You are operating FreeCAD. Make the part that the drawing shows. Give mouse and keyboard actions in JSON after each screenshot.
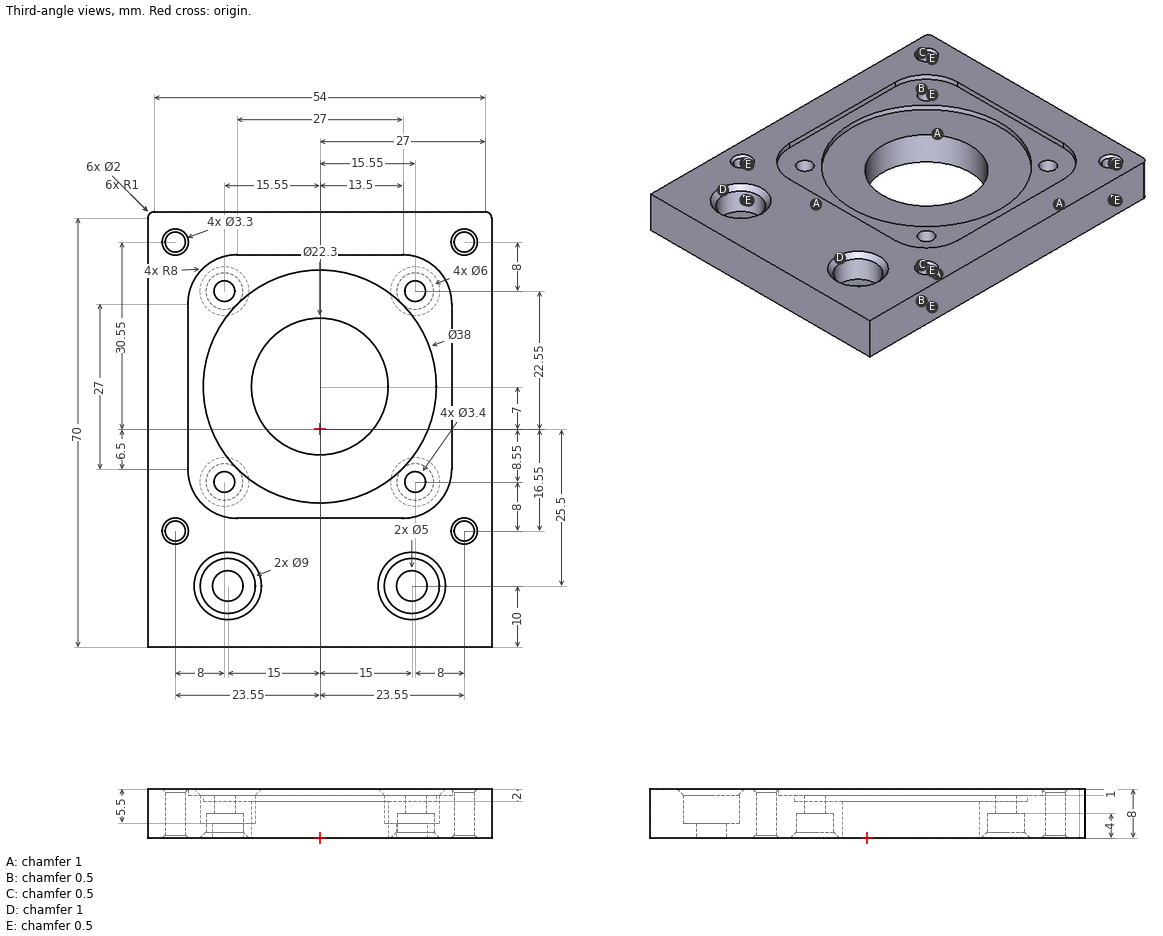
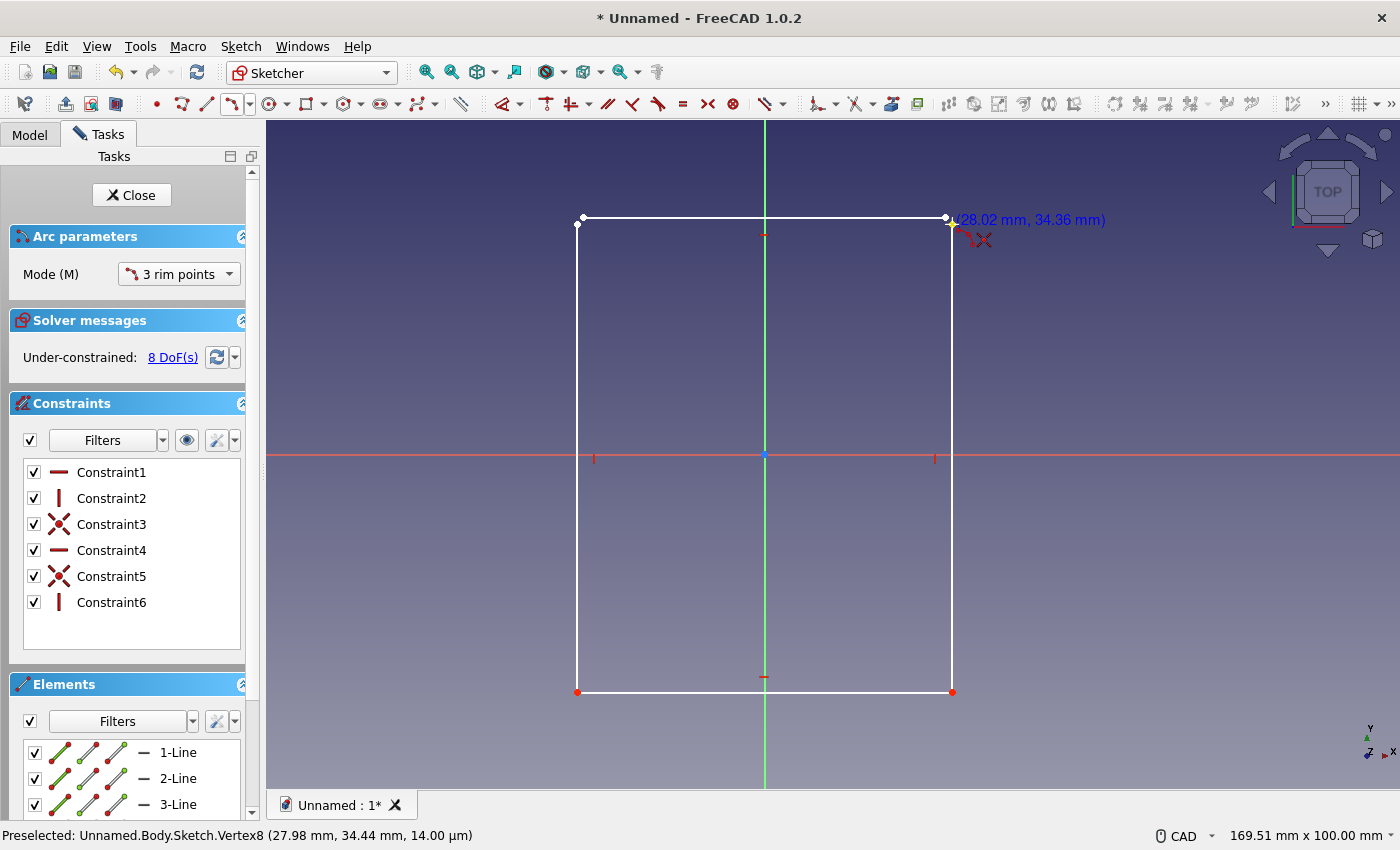
{"action": "scroll", "coordinate": [584, 217], "scroll_direction": "up", "scroll_amount": 3}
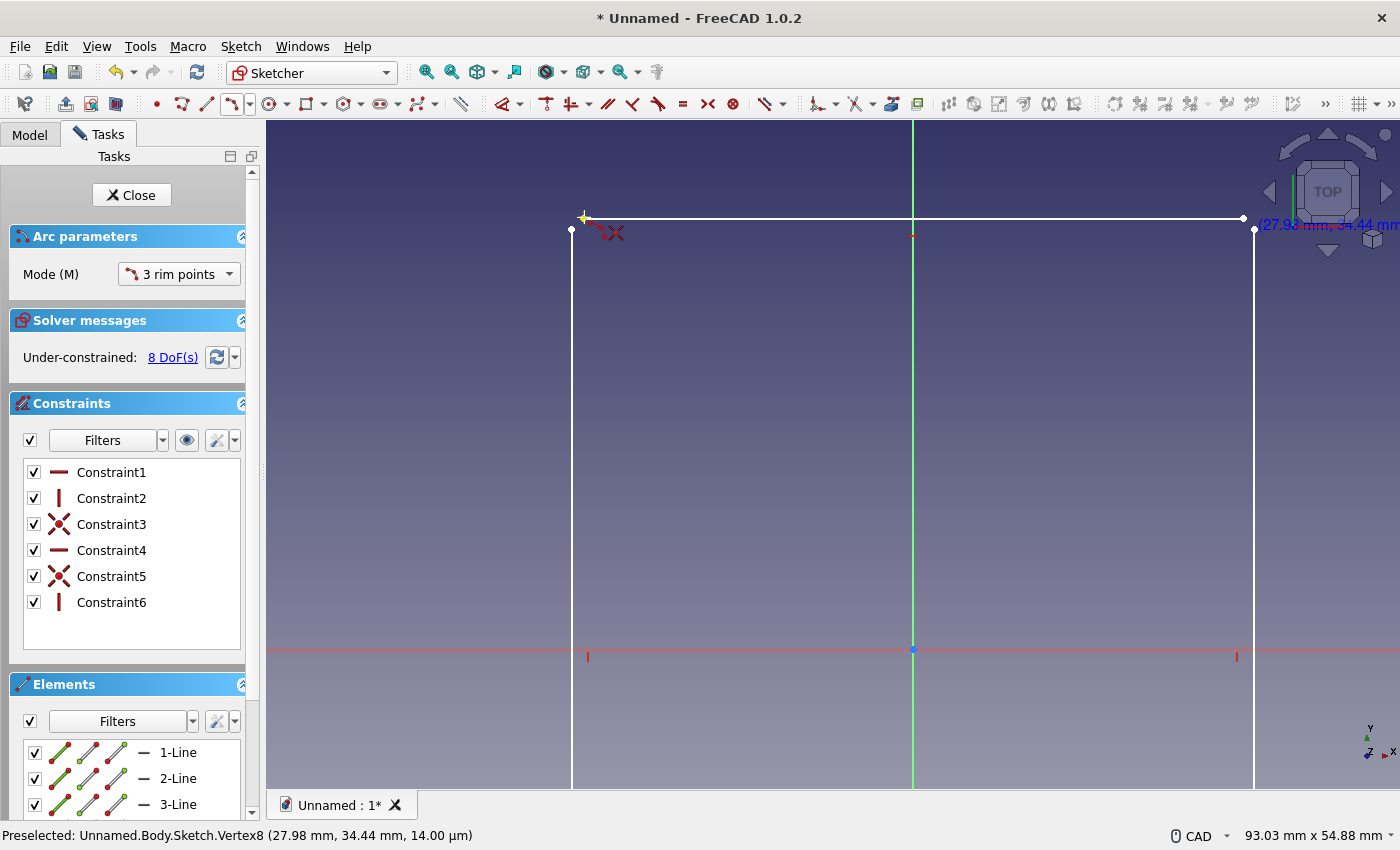
{"action": "left_click", "coordinate": [583, 219]}
{"action": "left_click", "coordinate": [572, 230]}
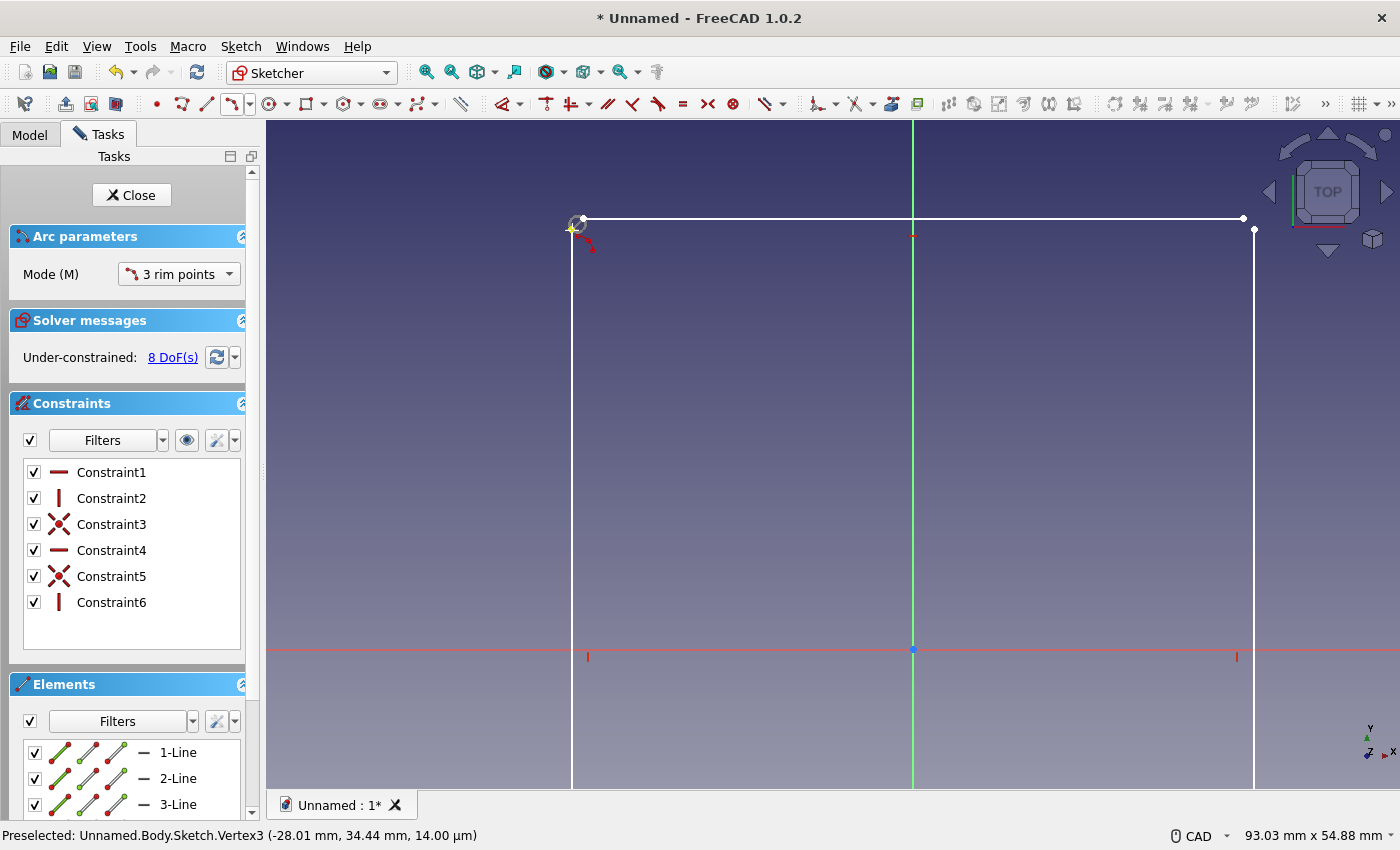
{"action": "scroll", "coordinate": [575, 220], "scroll_direction": "up", "scroll_amount": 8}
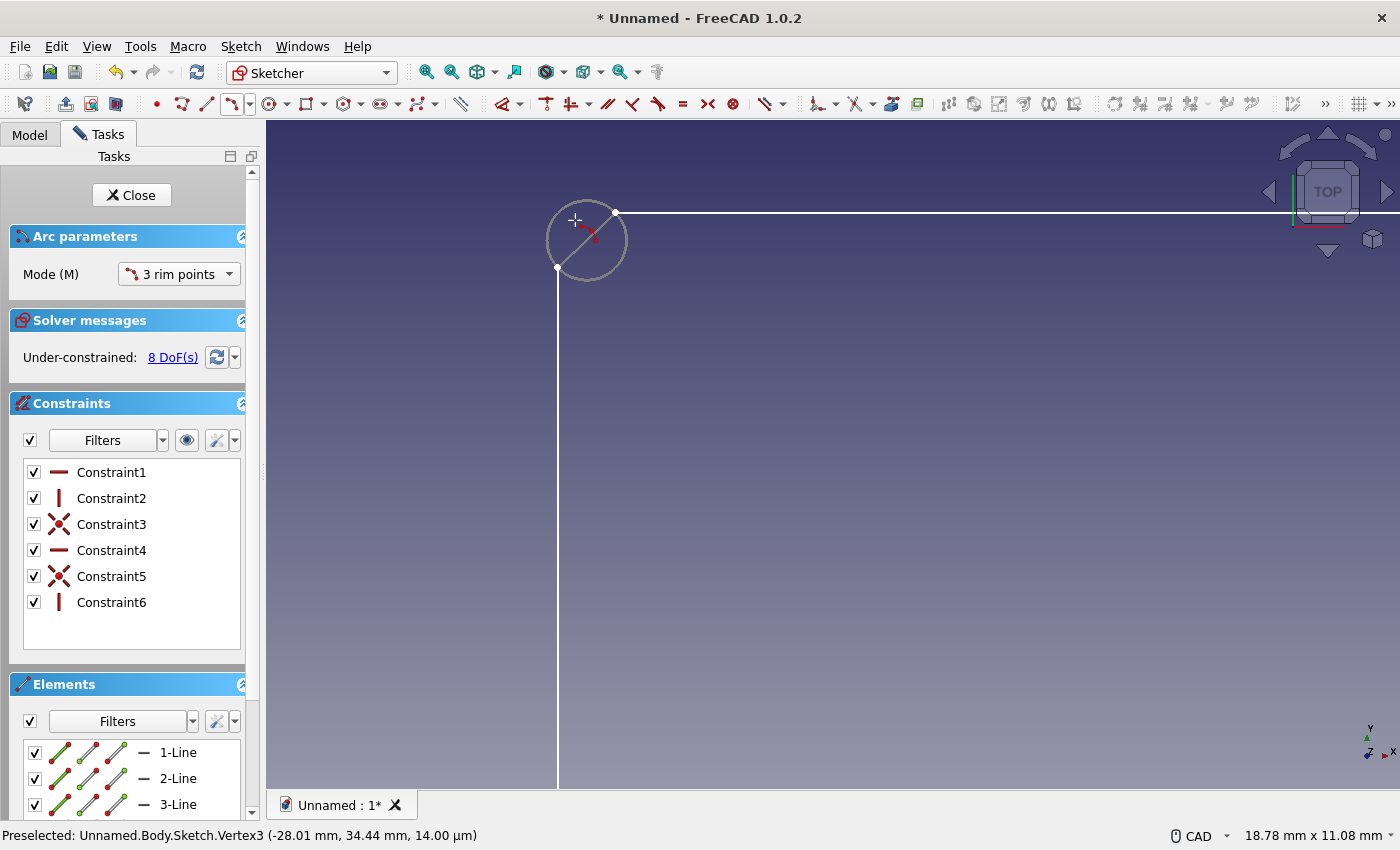
{"action": "left_click", "coordinate": [576, 222]}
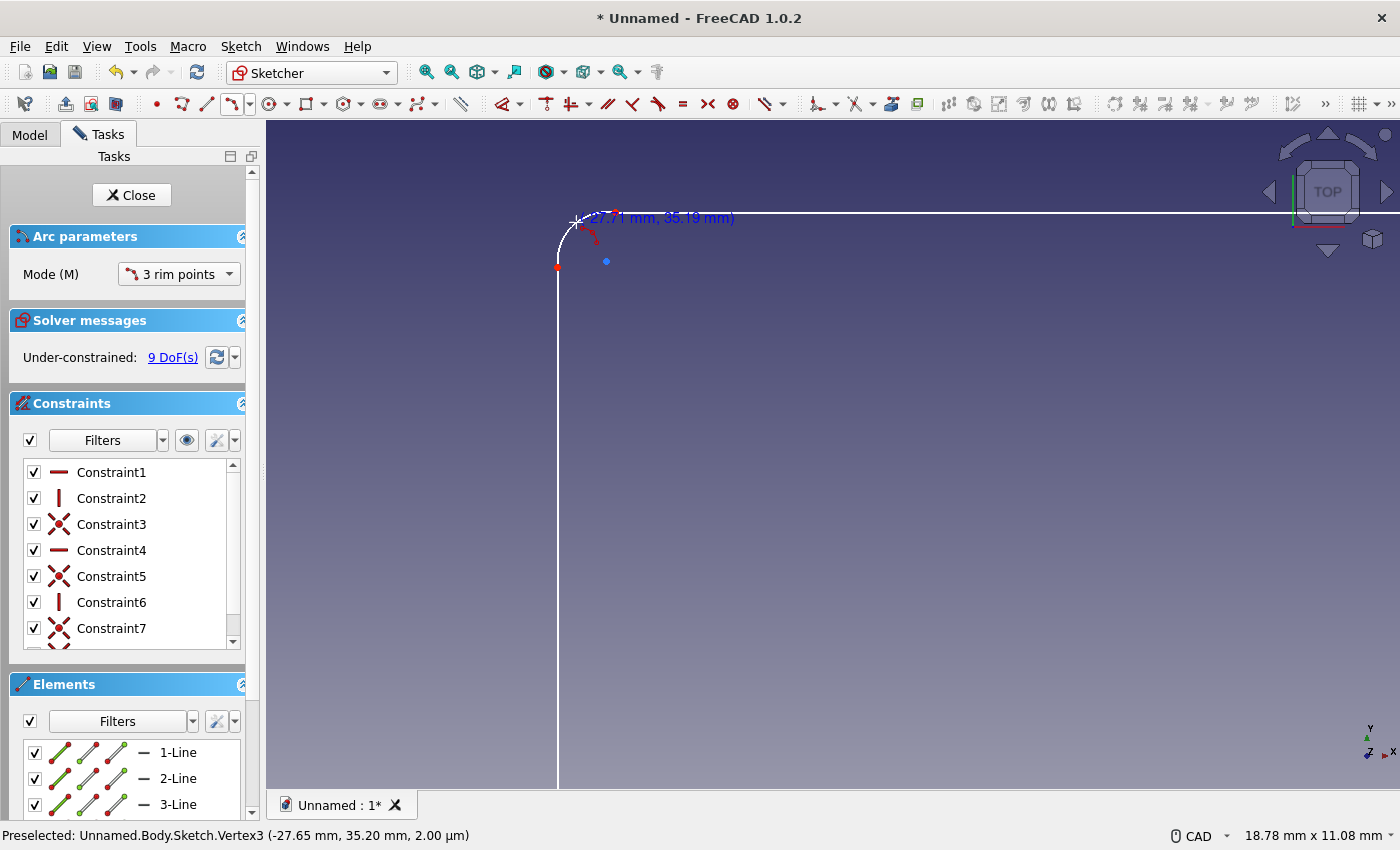
{"action": "scroll", "coordinate": [579, 219], "scroll_direction": "down", "scroll_amount": 11}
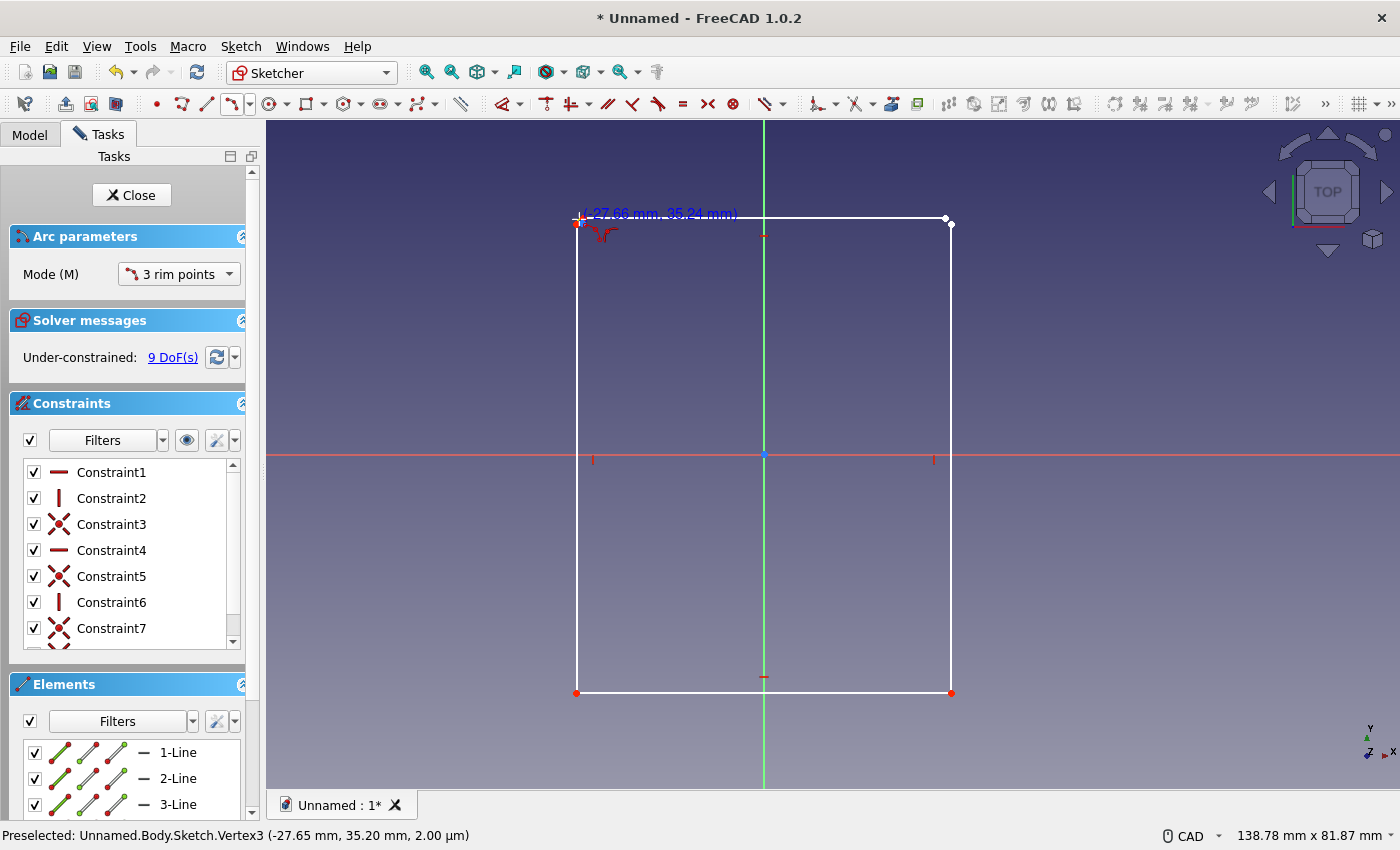
{"action": "scroll", "coordinate": [952, 224], "scroll_direction": "up", "scroll_amount": 3}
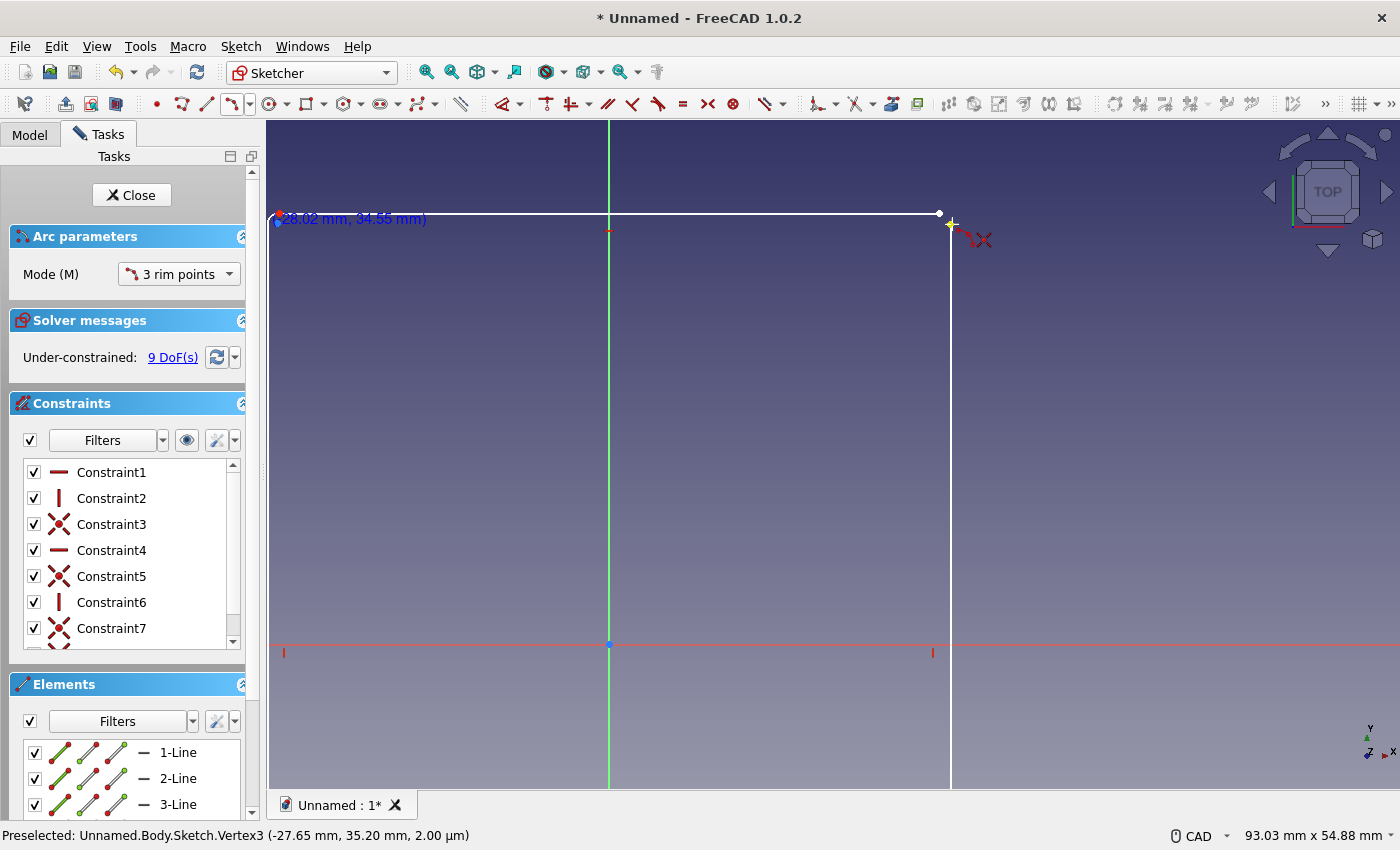
{"action": "left_click", "coordinate": [951, 225]}
{"action": "left_click", "coordinate": [939, 214]}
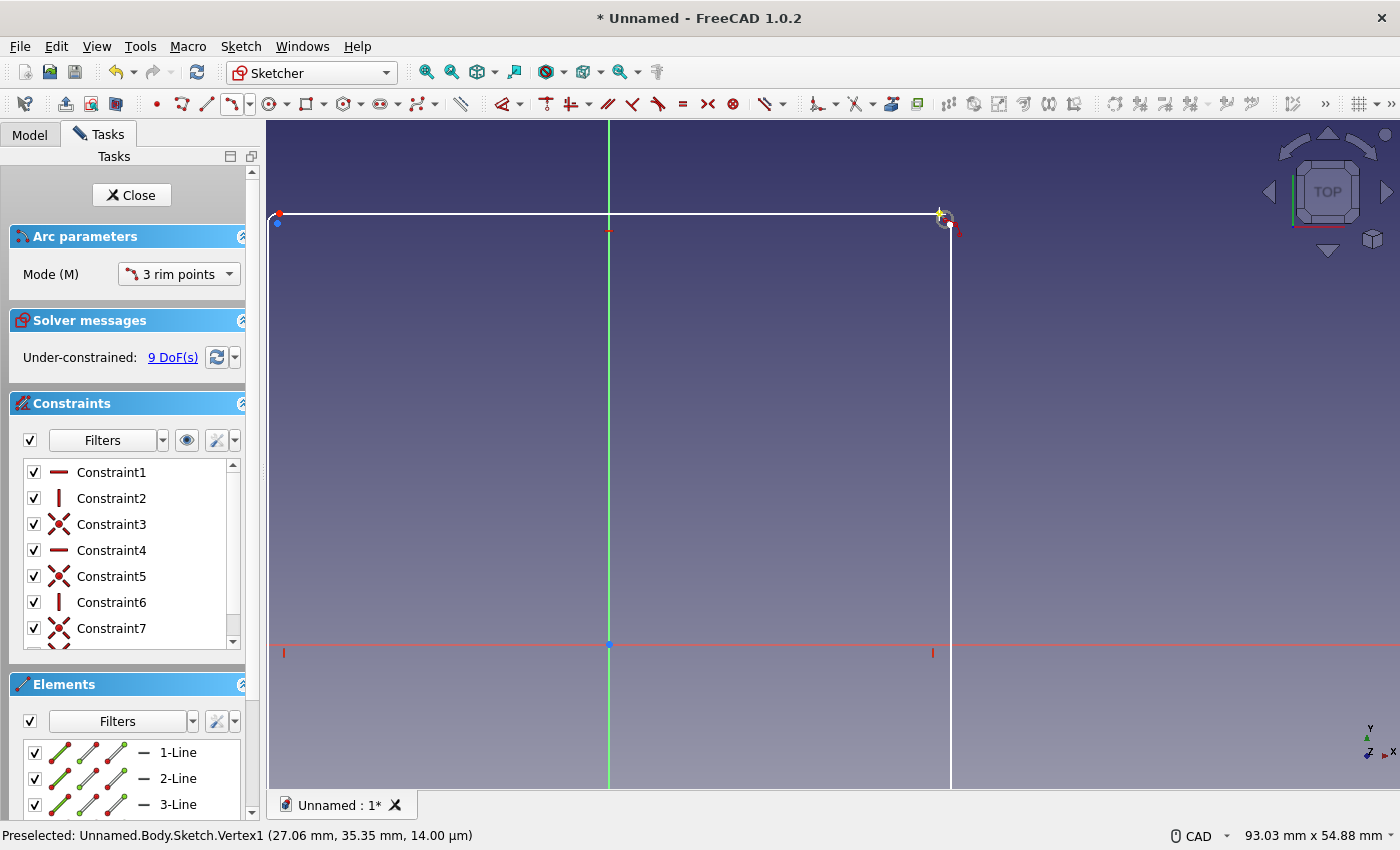
{"action": "scroll", "coordinate": [947, 216], "scroll_direction": "up", "scroll_amount": 8}